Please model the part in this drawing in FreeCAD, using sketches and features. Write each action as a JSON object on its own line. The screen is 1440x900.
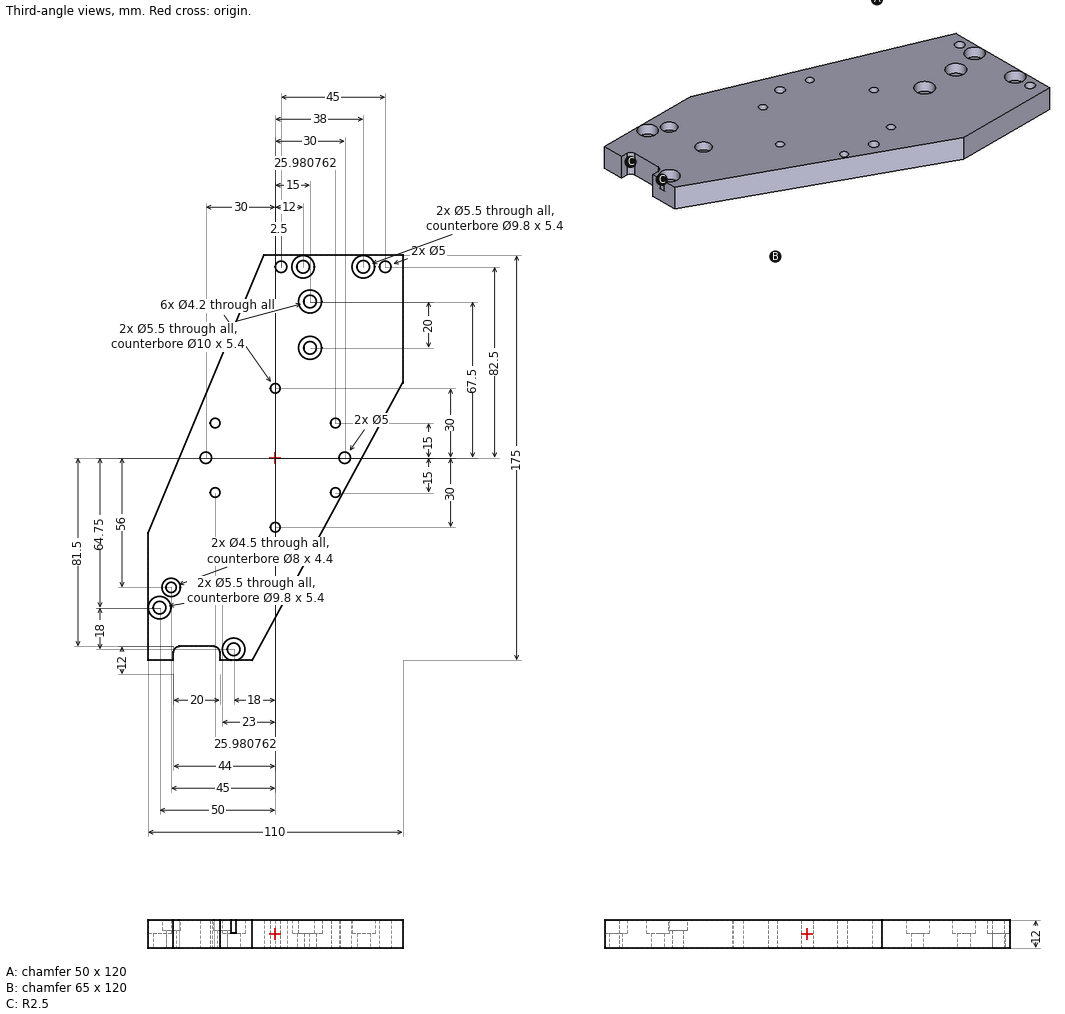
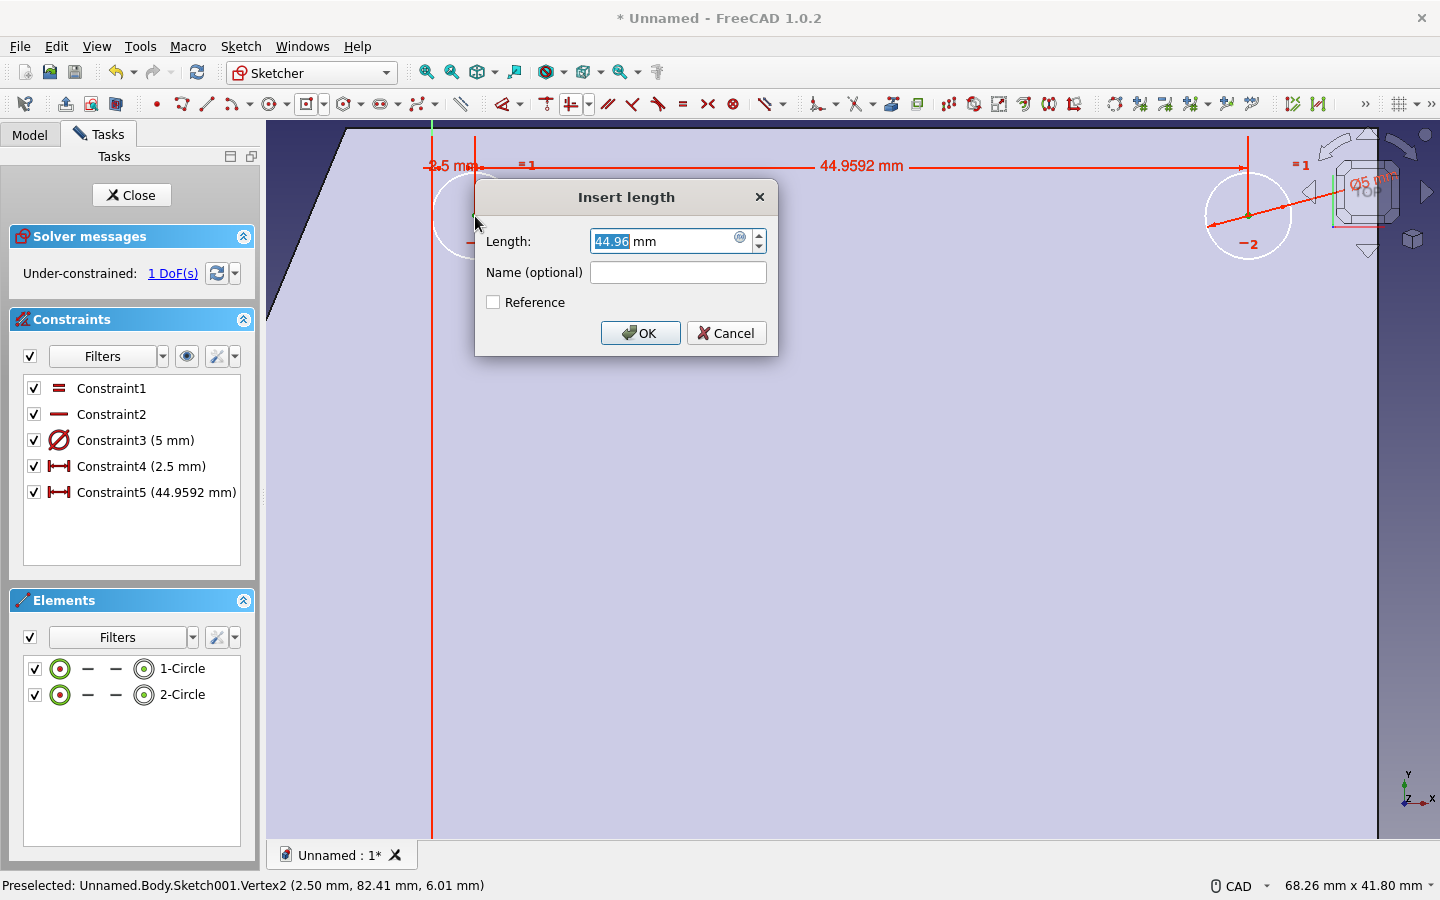
{"action": "type", "text": "45"}
{"action": "key", "text": "Return"}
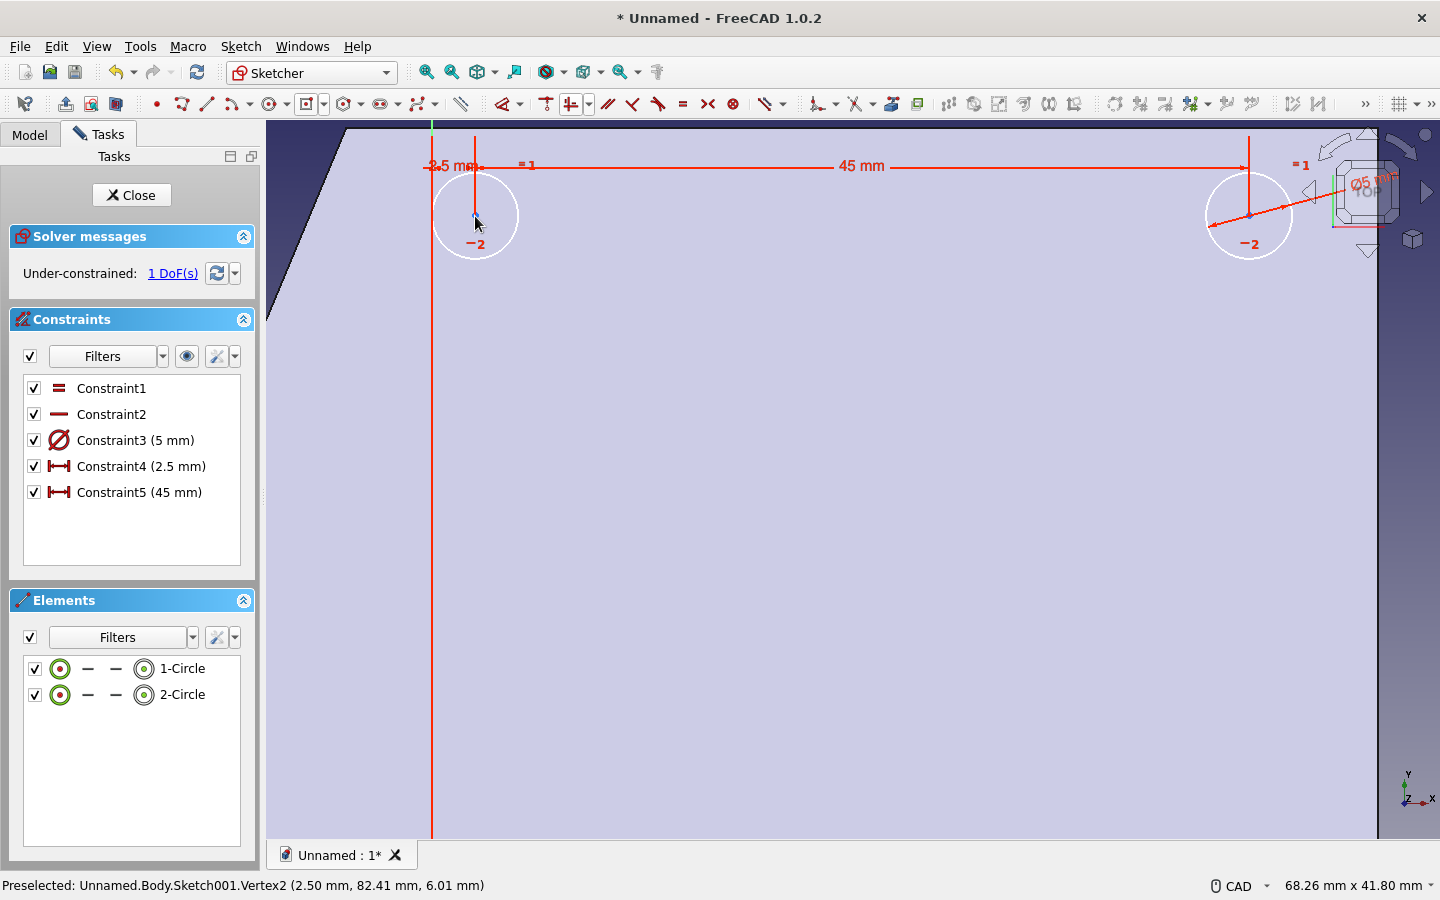
{"action": "left_click", "coordinate": [1249, 216]}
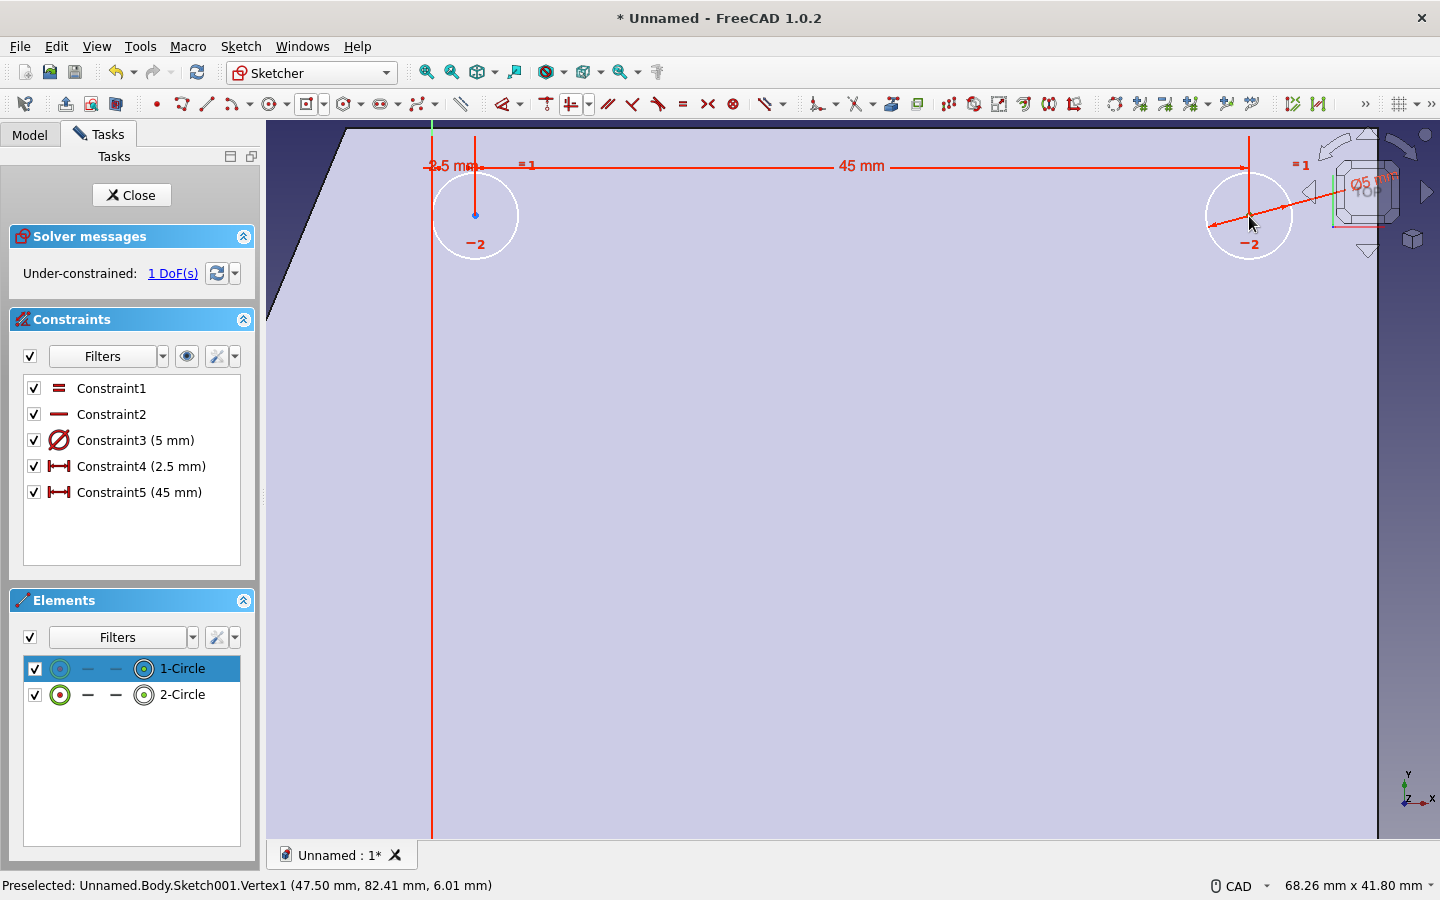
{"action": "key", "text": "i"}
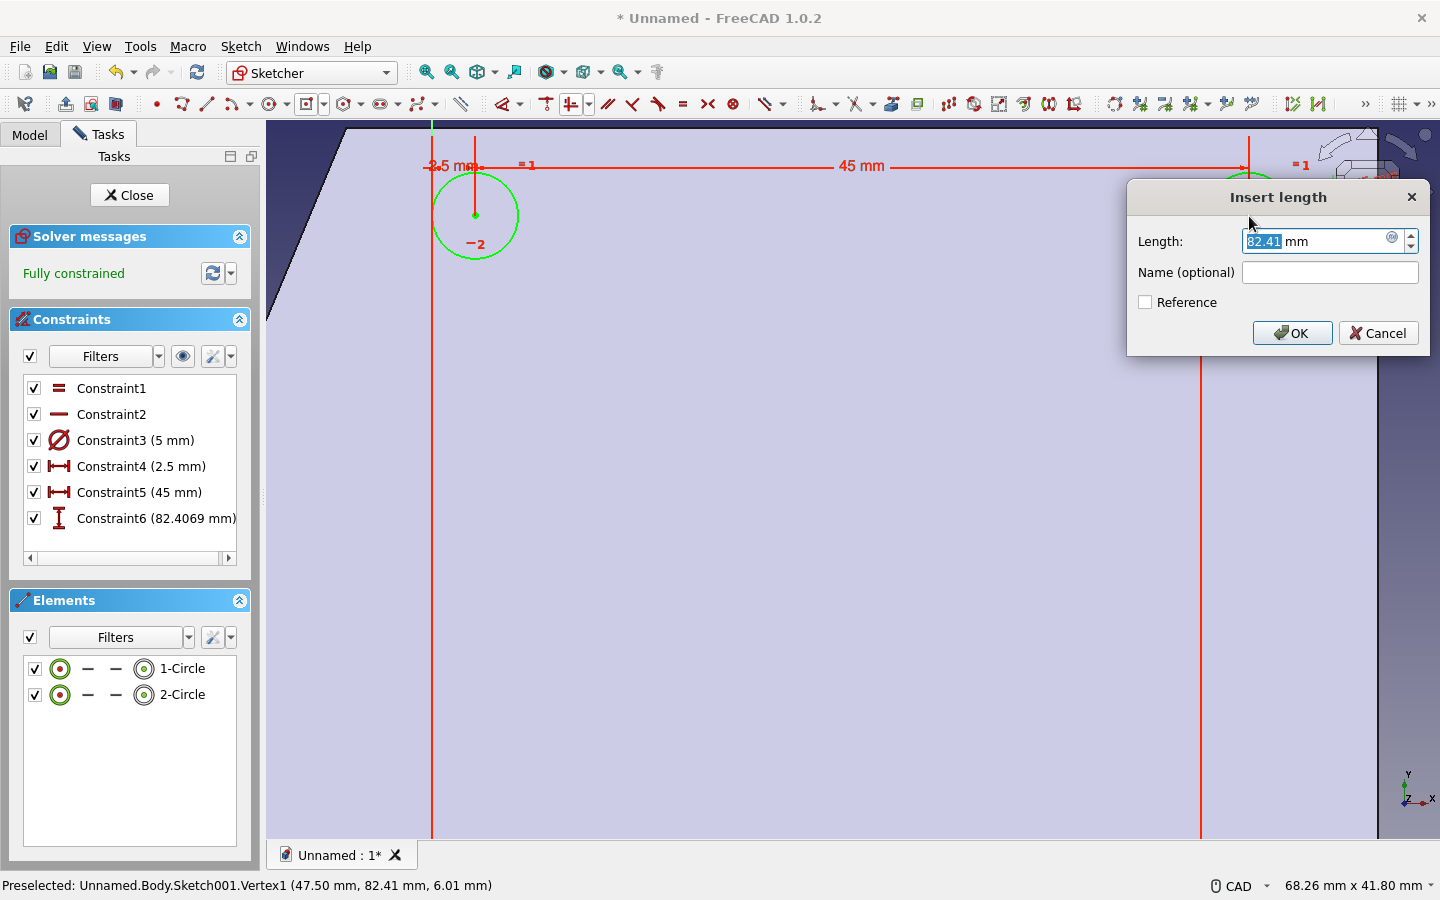
{"action": "type", "text": "82.5"}
{"action": "key", "text": "Return"}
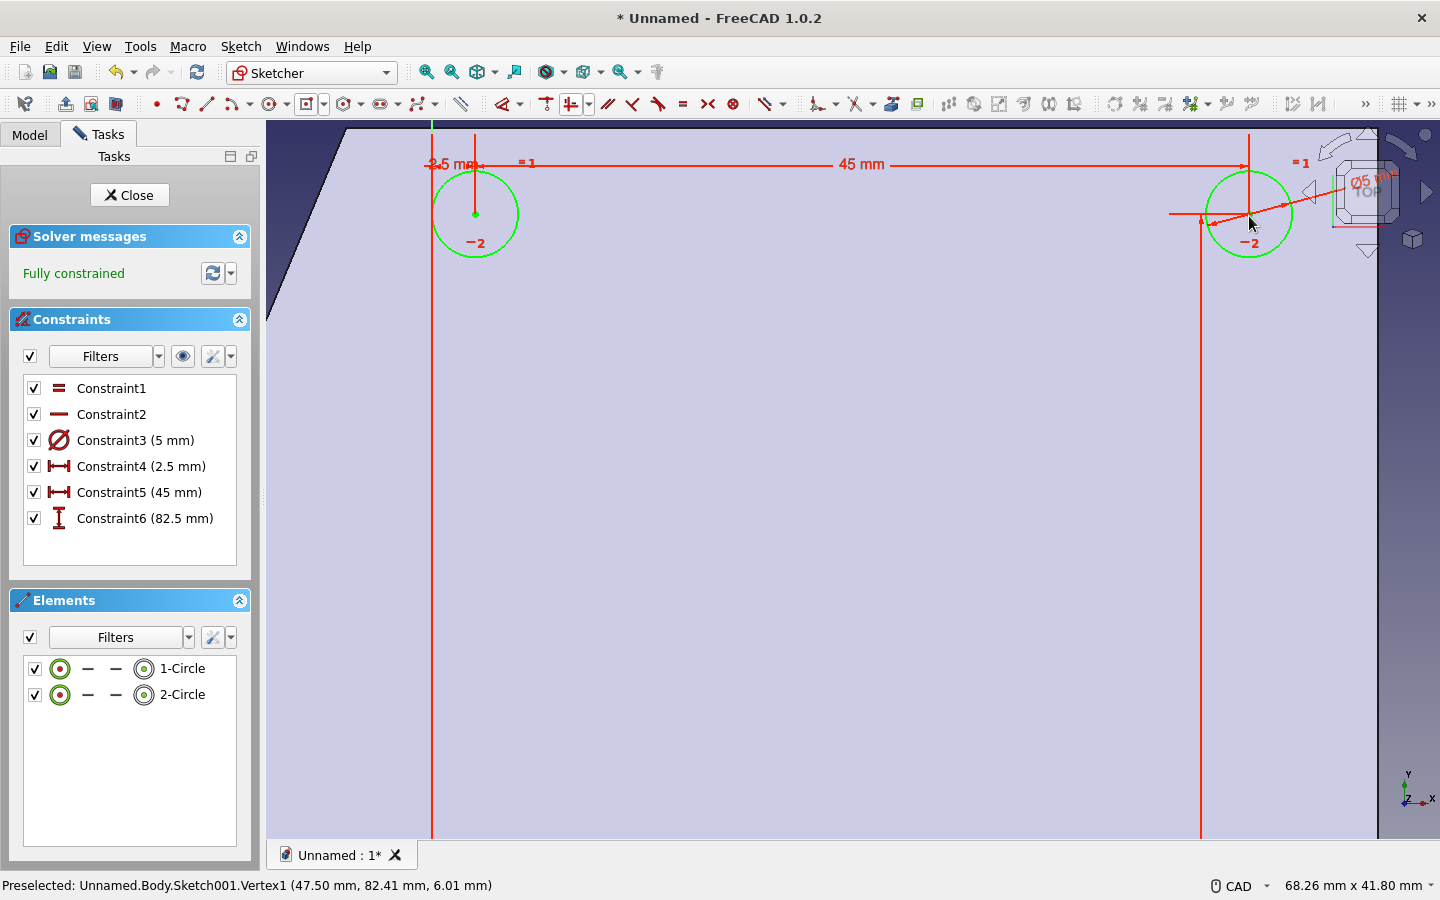
{"action": "left_click", "coordinate": [130, 195]}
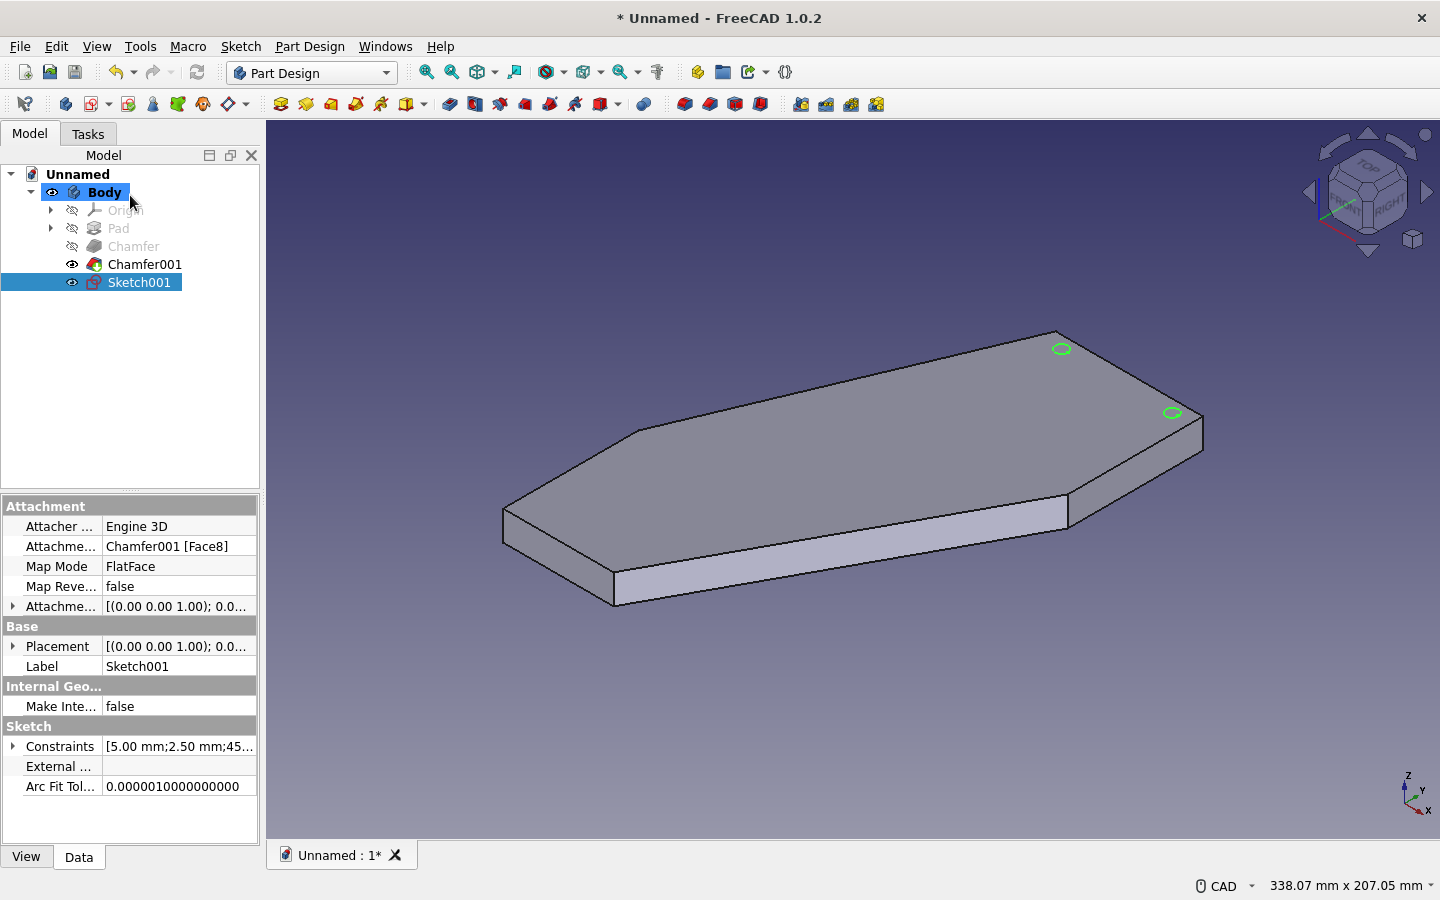
{"action": "left_click", "coordinate": [450, 104]}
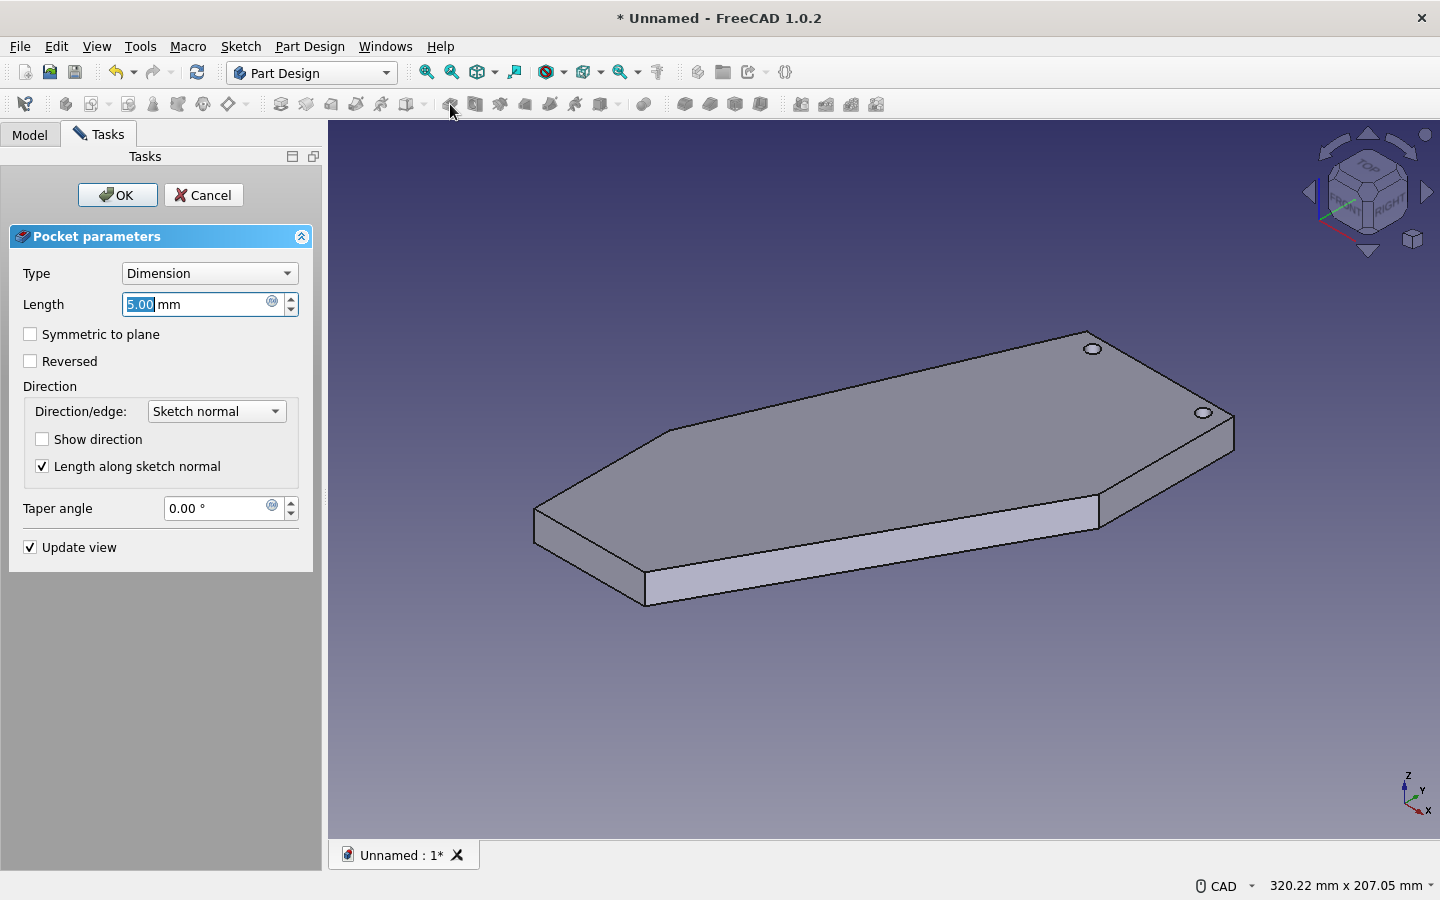
{"action": "left_click", "coordinate": [210, 274]}